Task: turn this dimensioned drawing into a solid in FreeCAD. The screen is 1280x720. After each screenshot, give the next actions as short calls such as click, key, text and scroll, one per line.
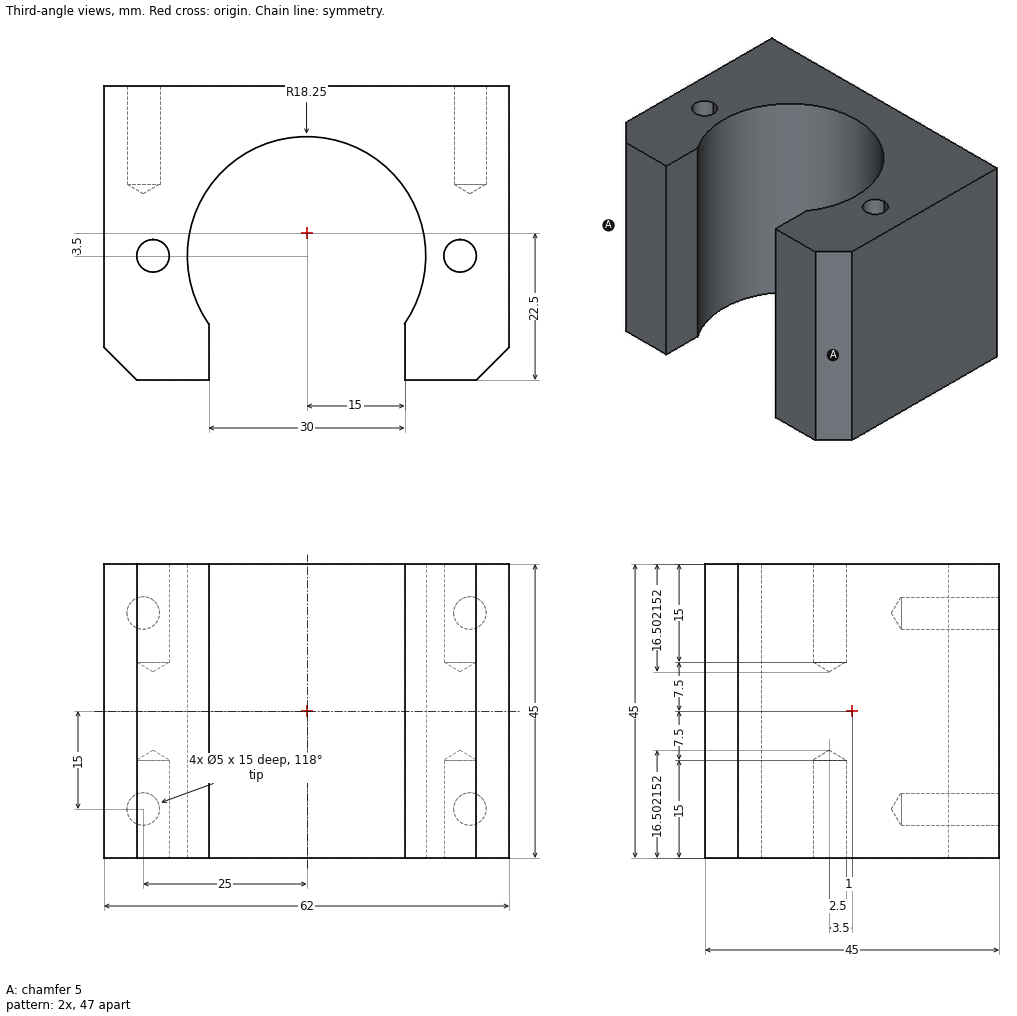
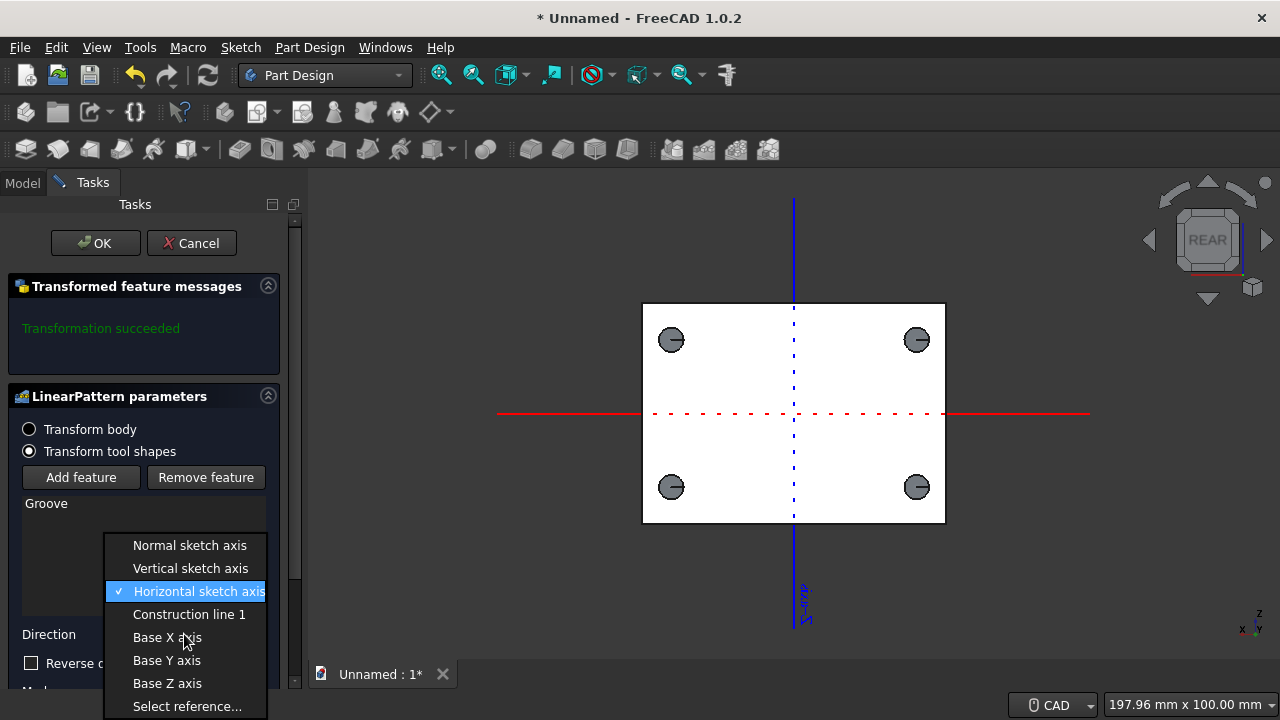
click(184, 638)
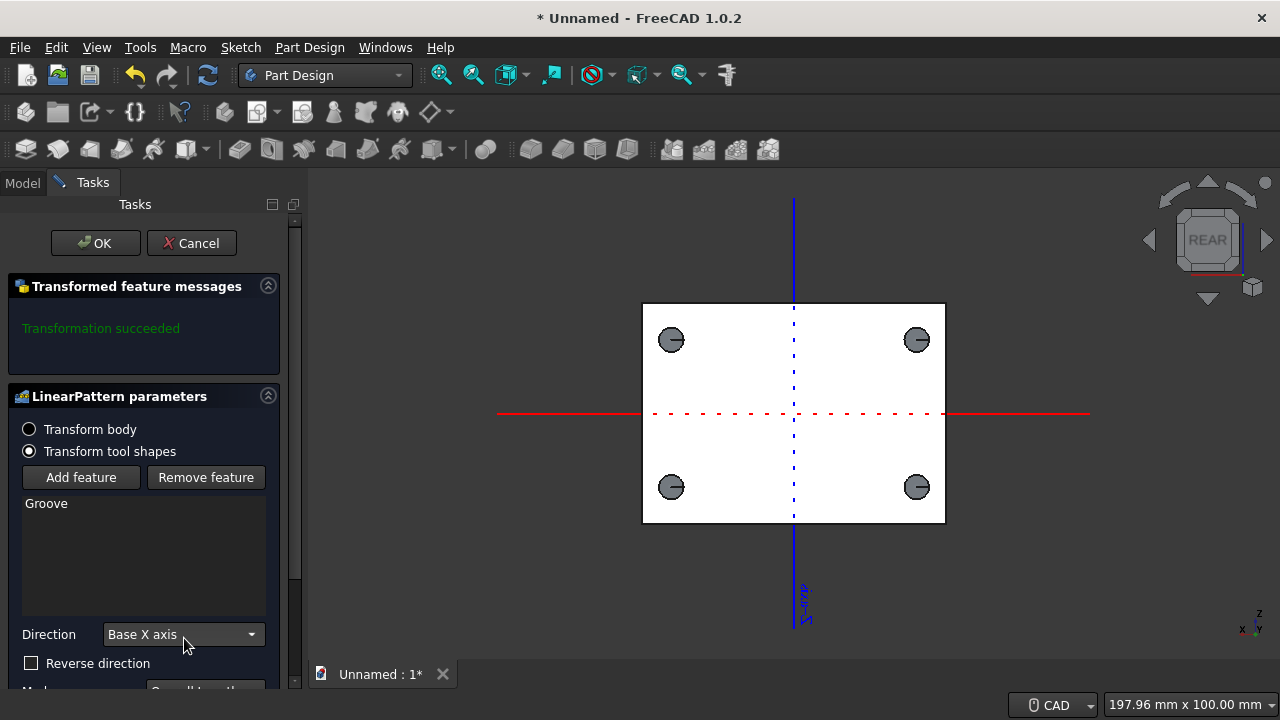
scroll(295, 451, down, 2)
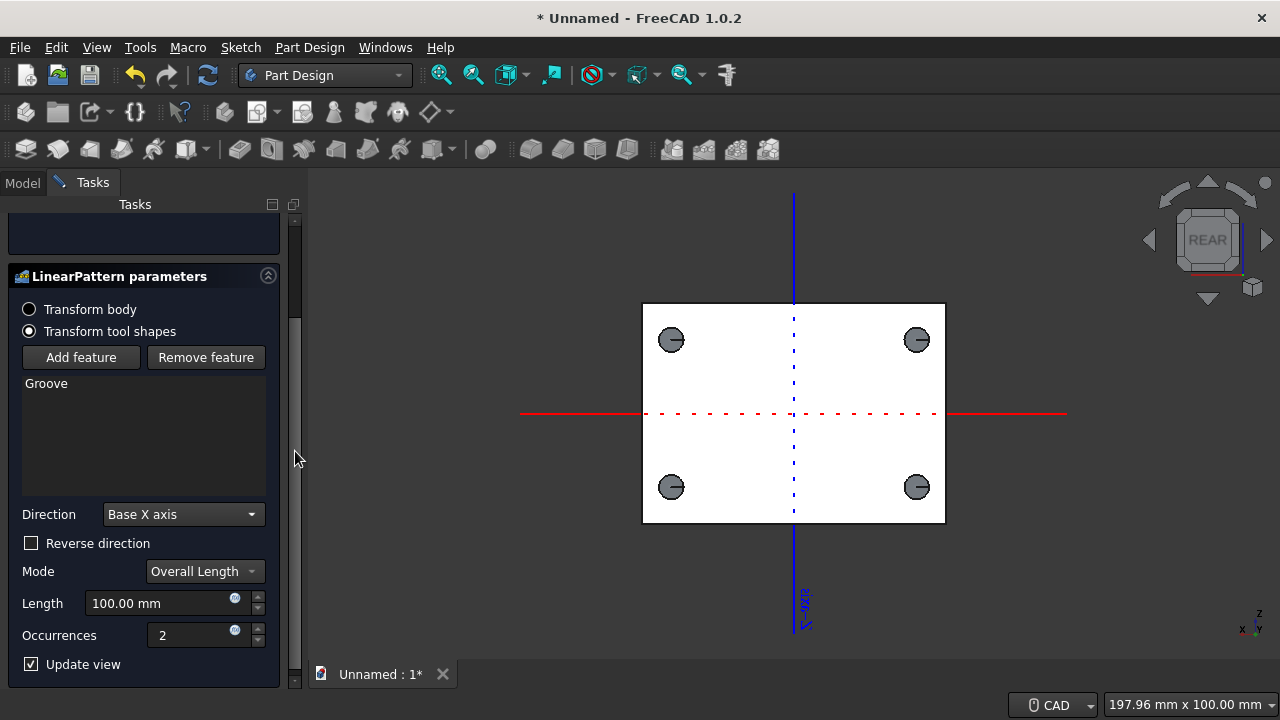
click(206, 572)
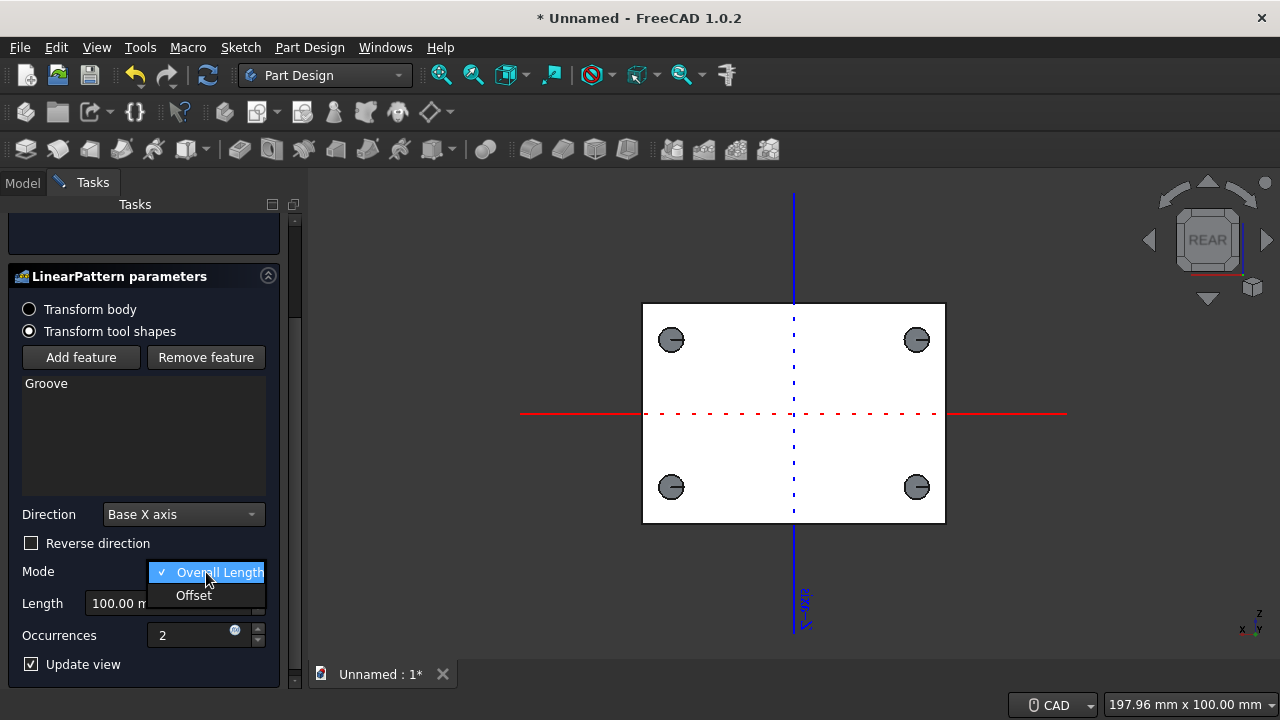
click(206, 596)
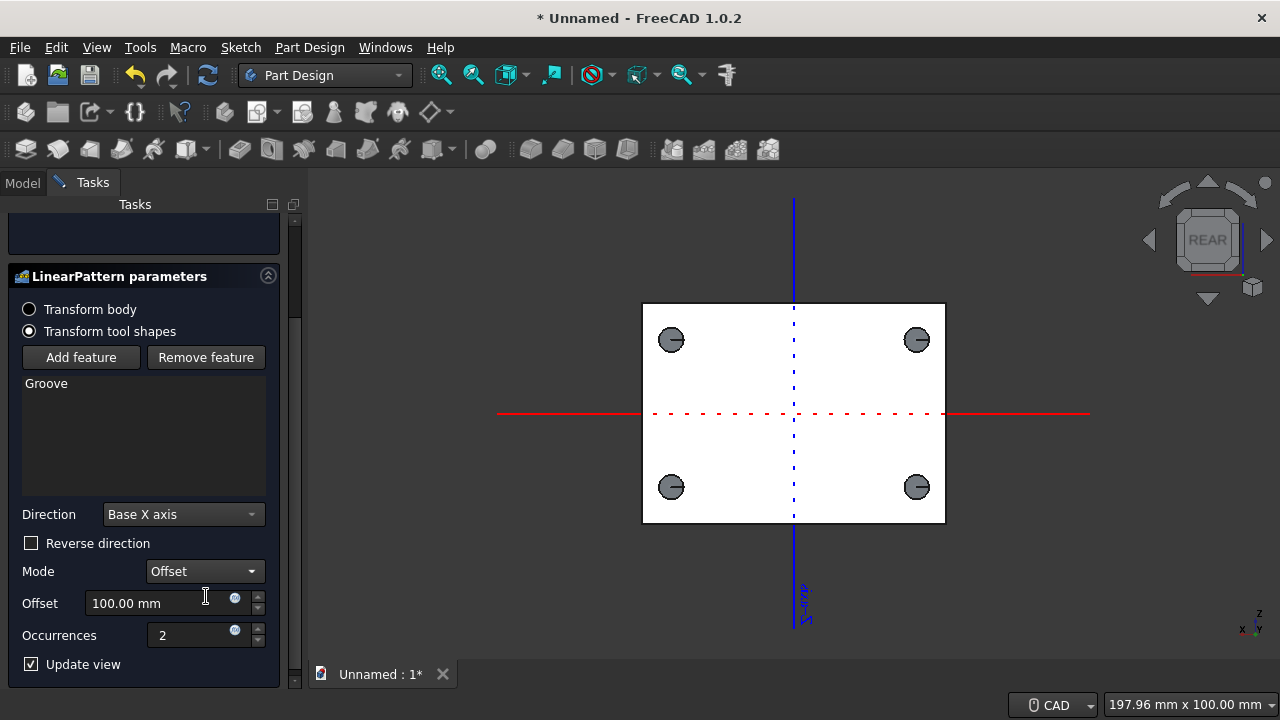
triple_click(168, 603)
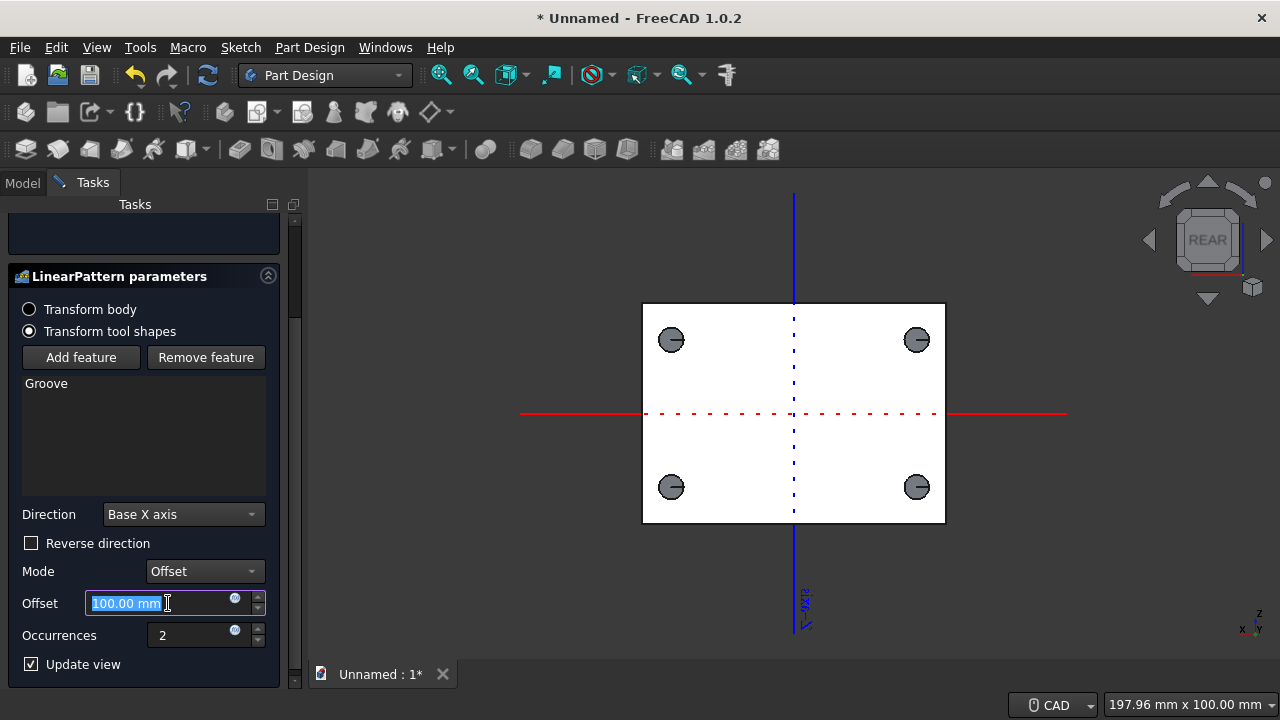
text(47)
key(Tab)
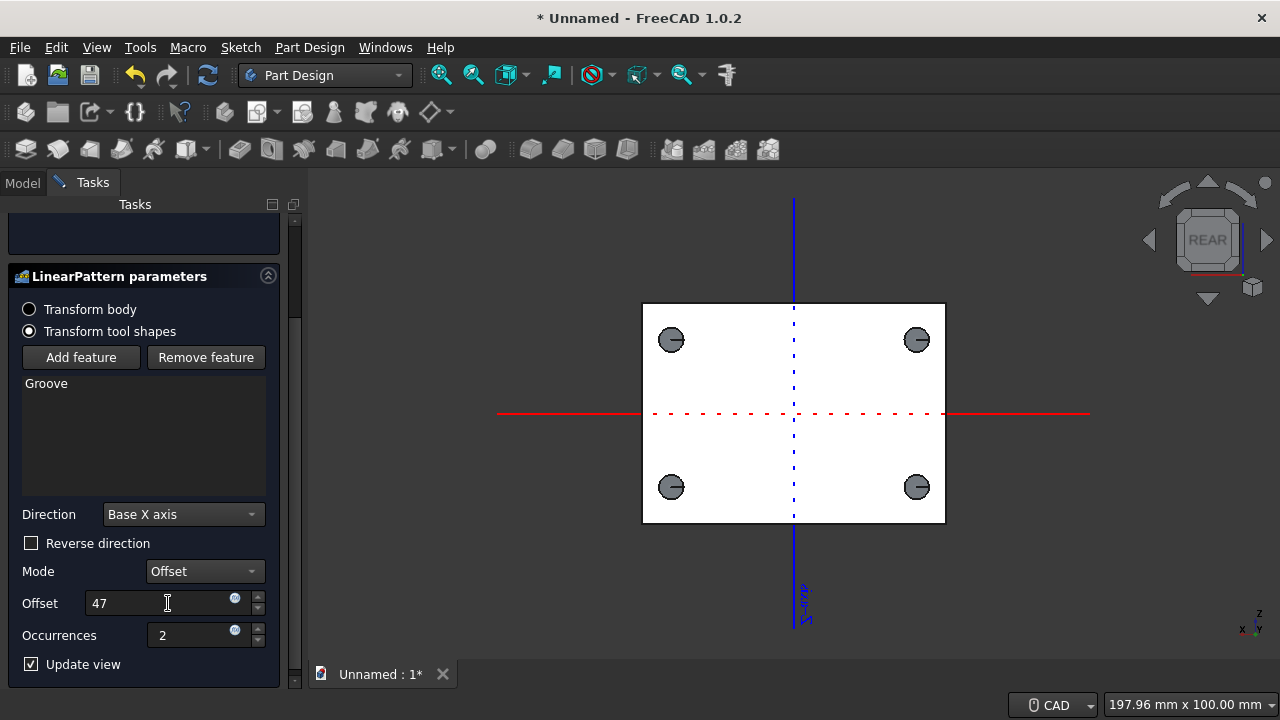
triple_click(198, 635)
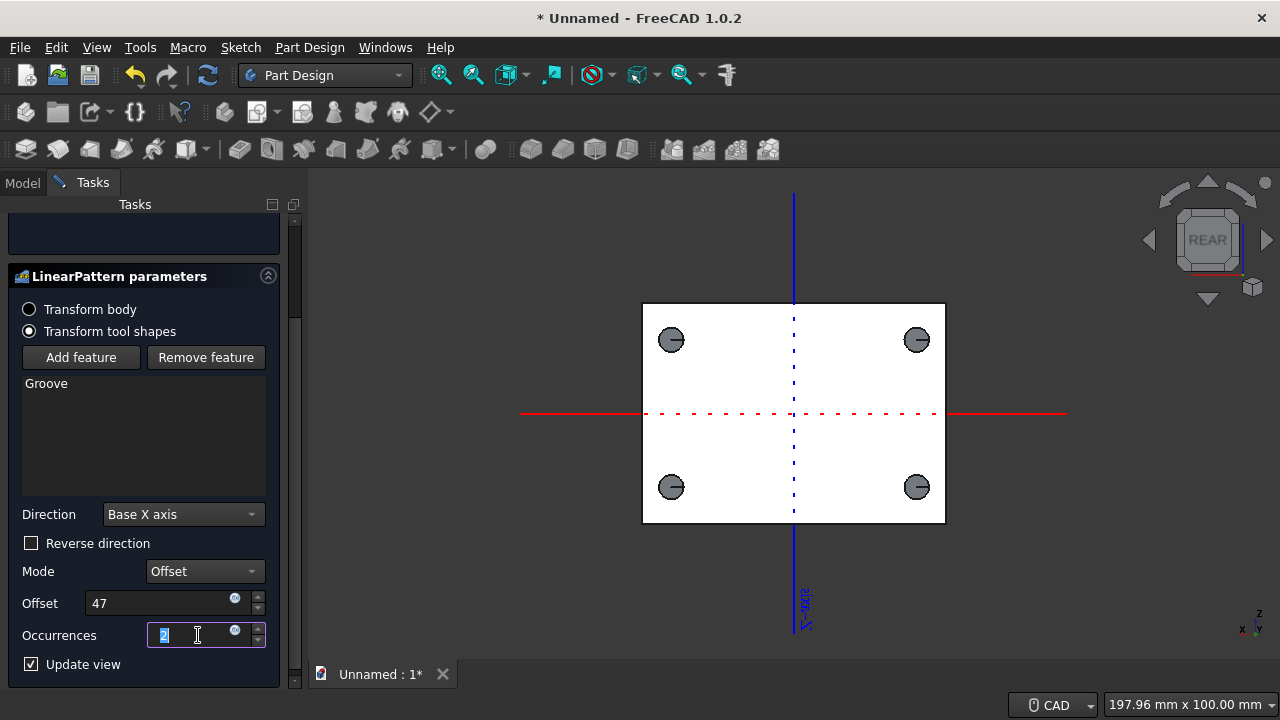
text(2)
key(Tab)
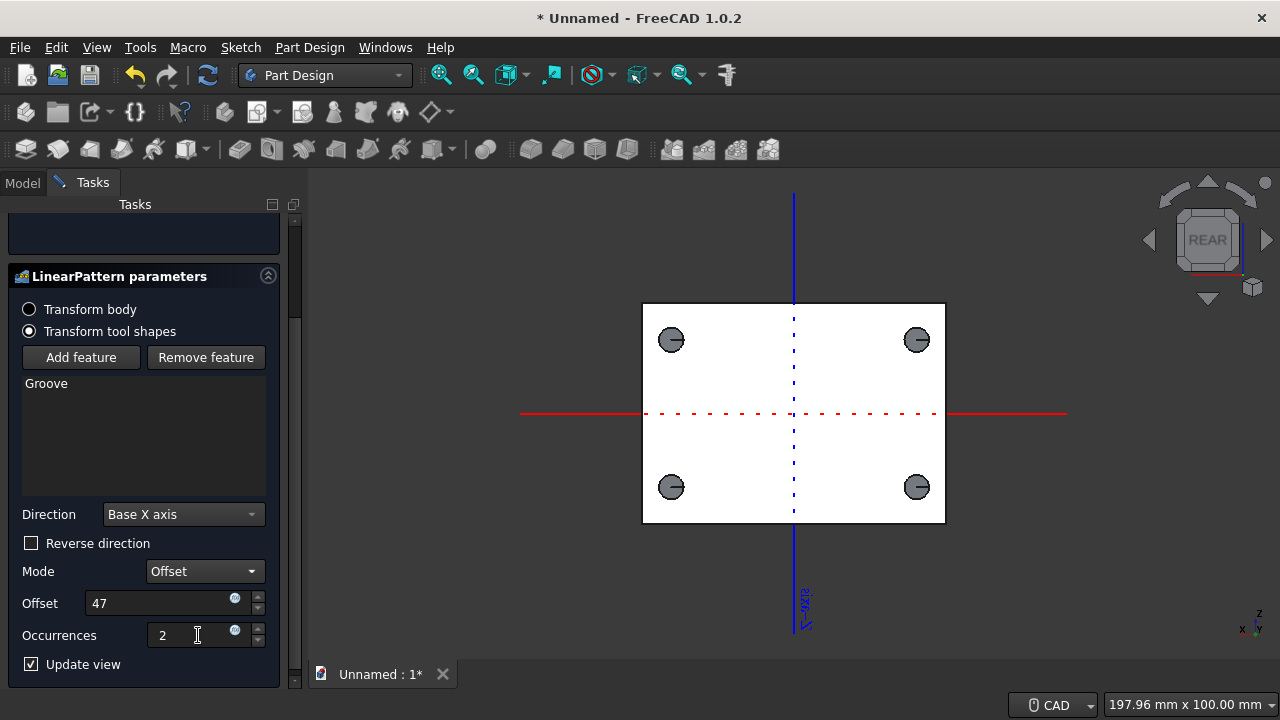
click(30, 543)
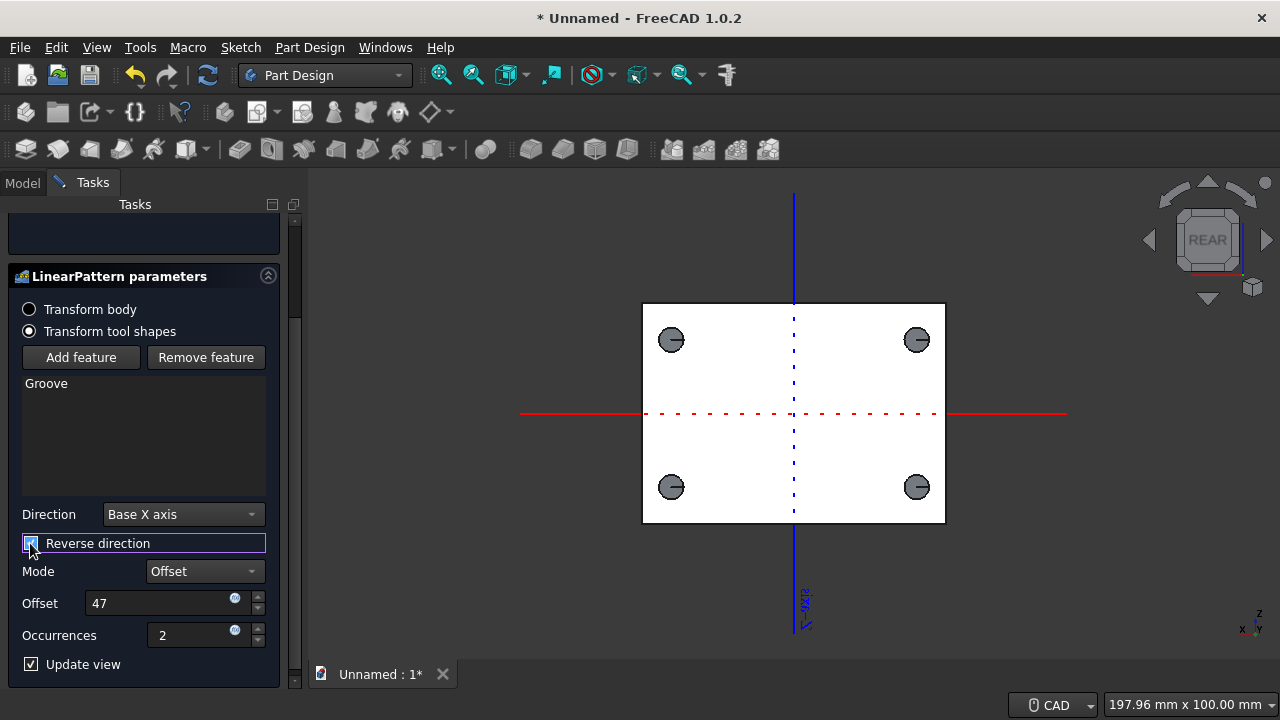
scroll(295, 451, up, 3)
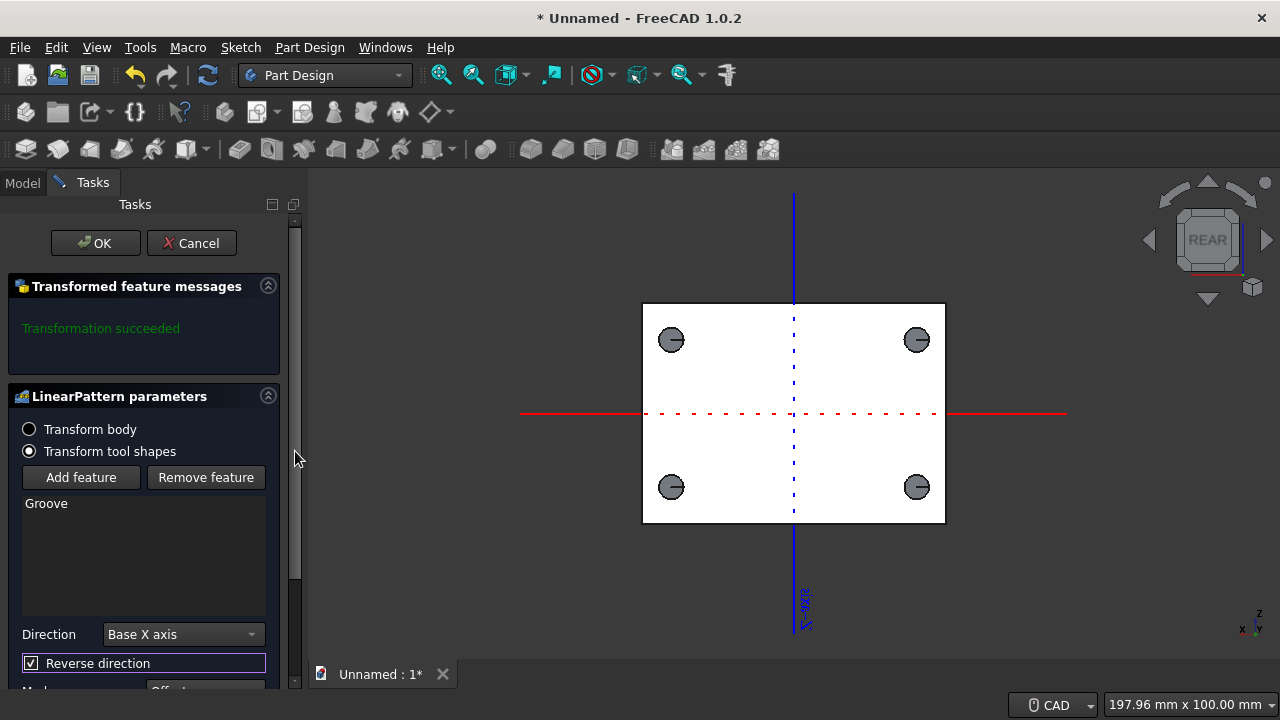
click(96, 243)